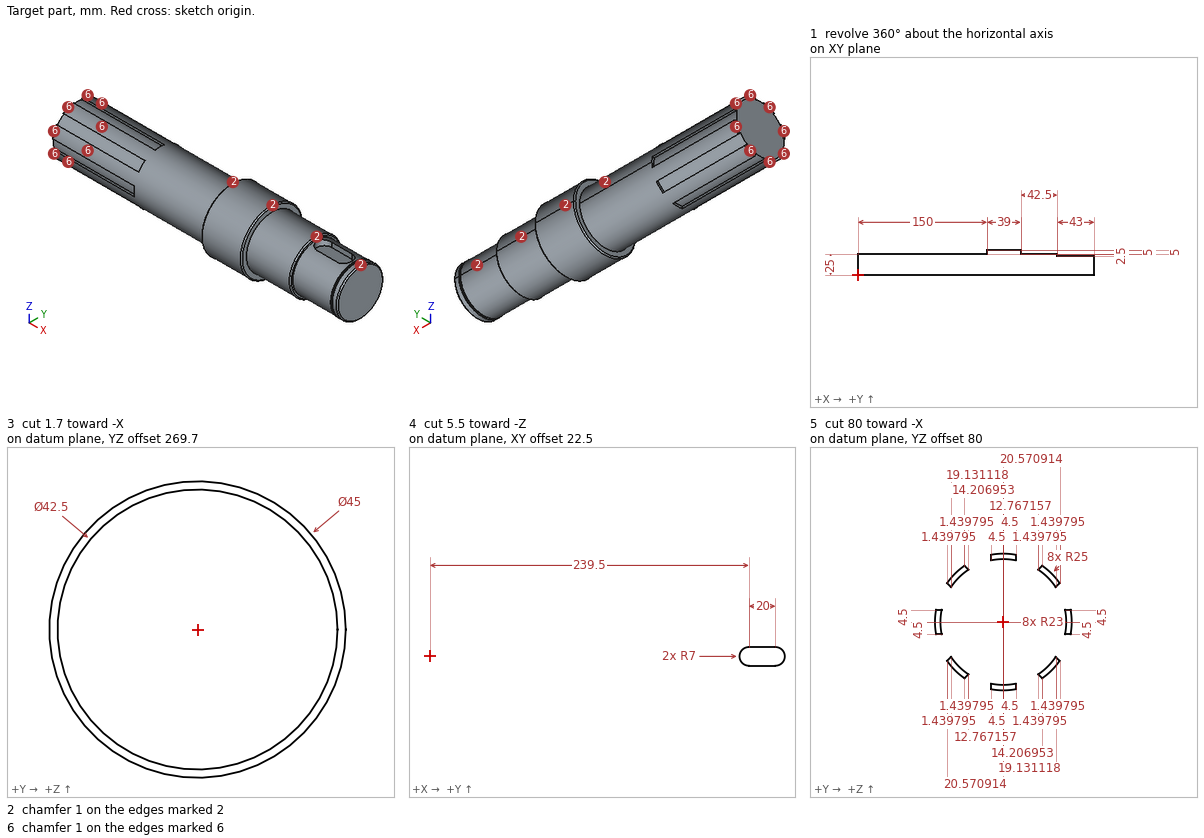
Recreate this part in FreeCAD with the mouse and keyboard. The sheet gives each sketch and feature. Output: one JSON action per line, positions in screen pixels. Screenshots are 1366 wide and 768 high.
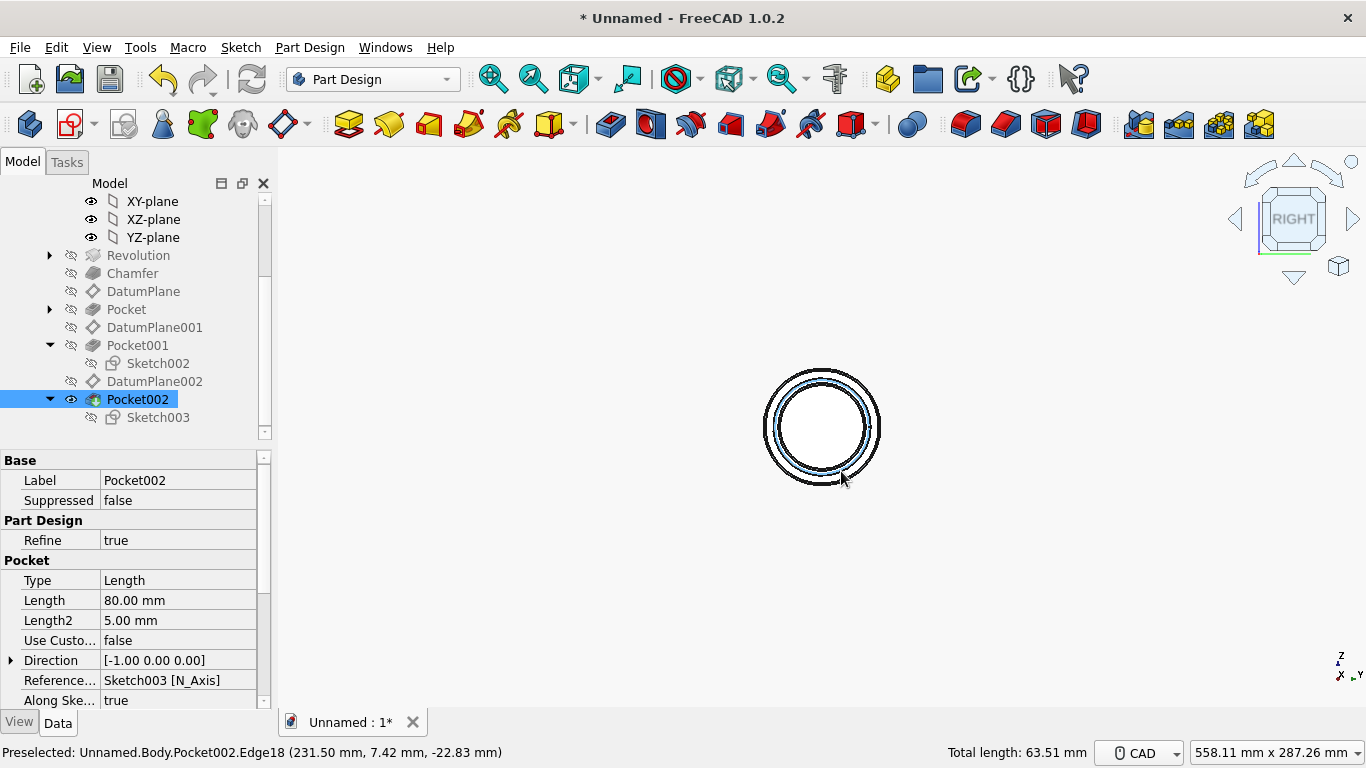
{"action": "key", "text": "5"}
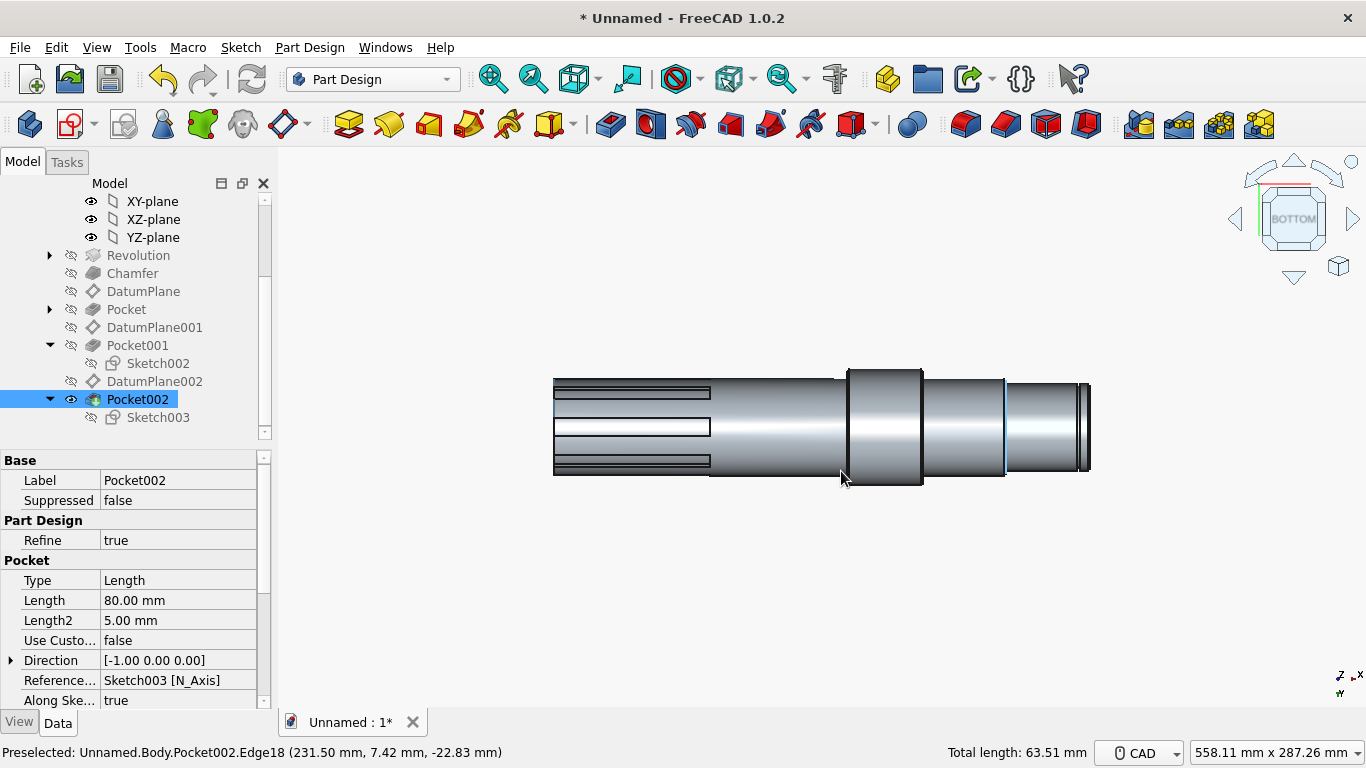
{"action": "left_click", "coordinate": [554, 445], "text": "ctrl"}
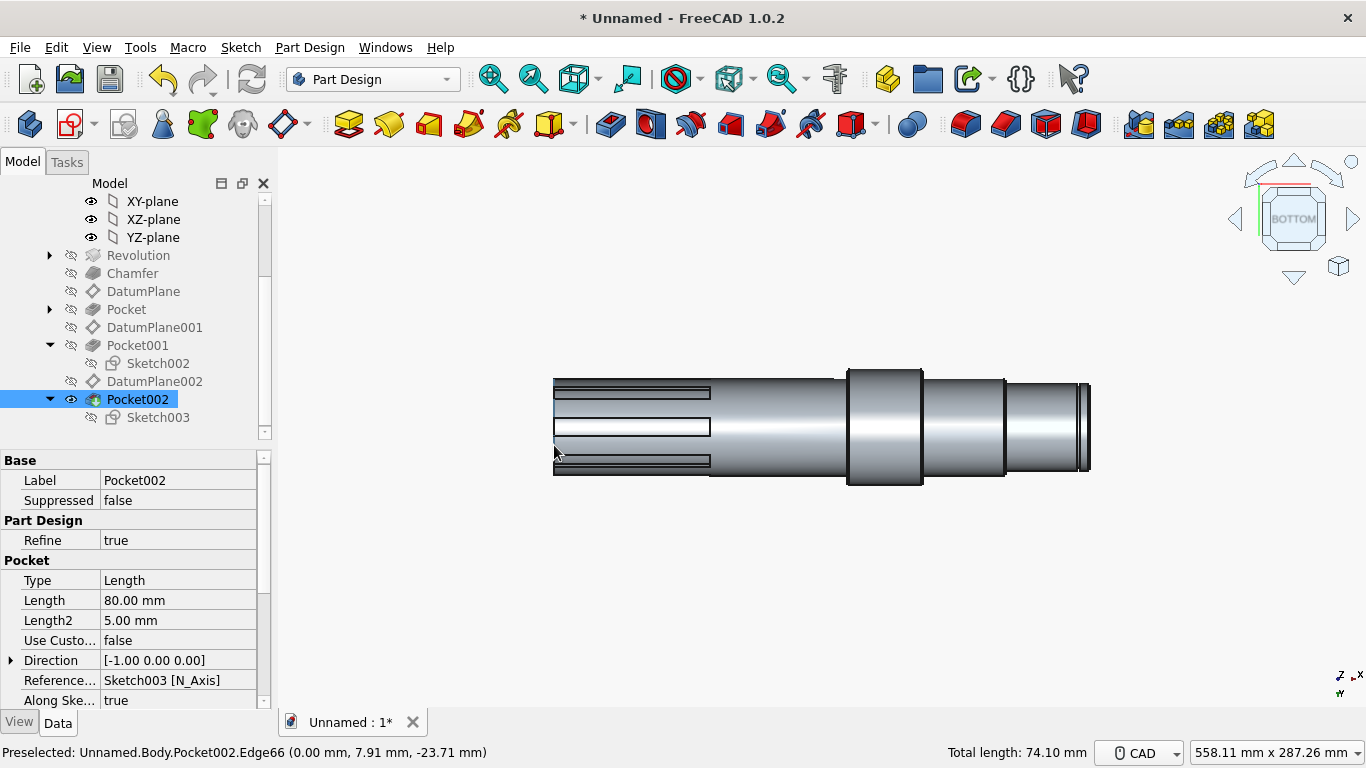
{"action": "left_click", "coordinate": [554, 473], "text": "ctrl"}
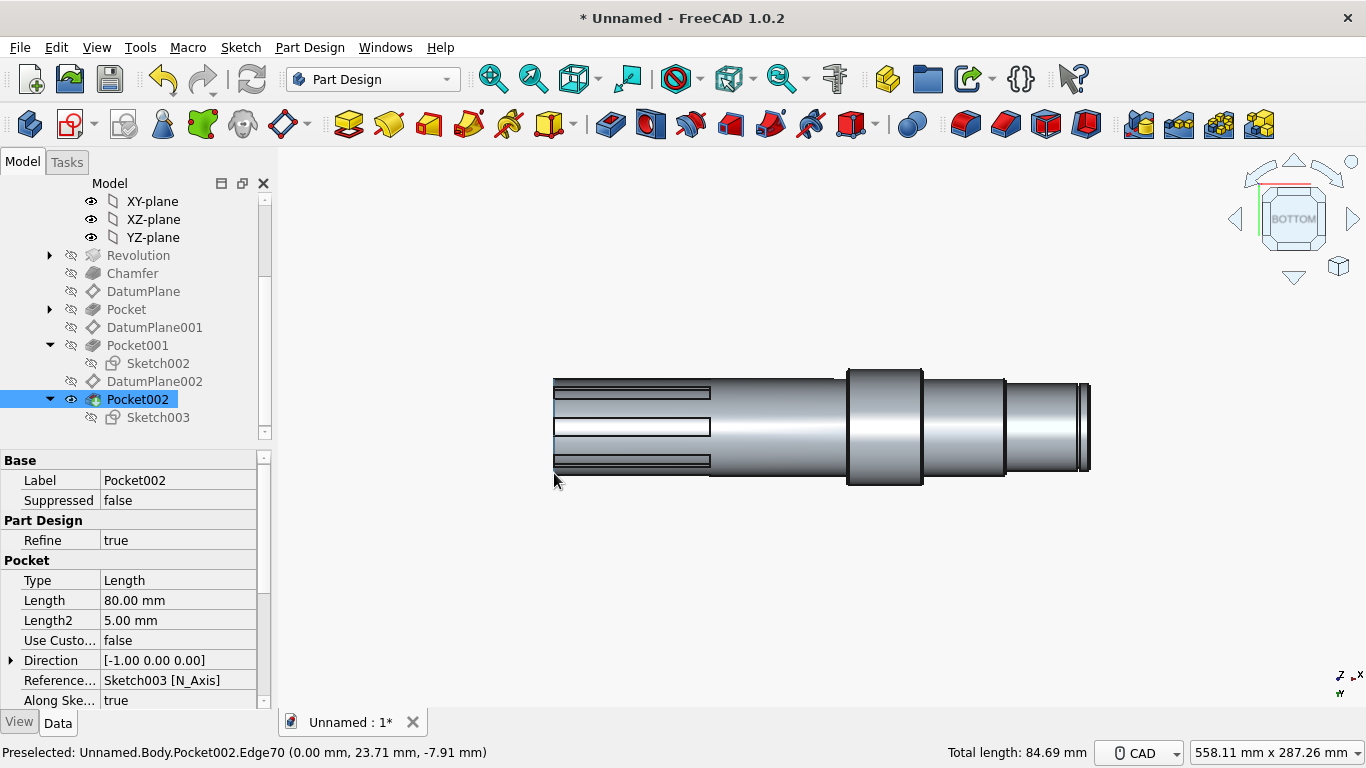
{"action": "left_click", "coordinate": [1006, 124]}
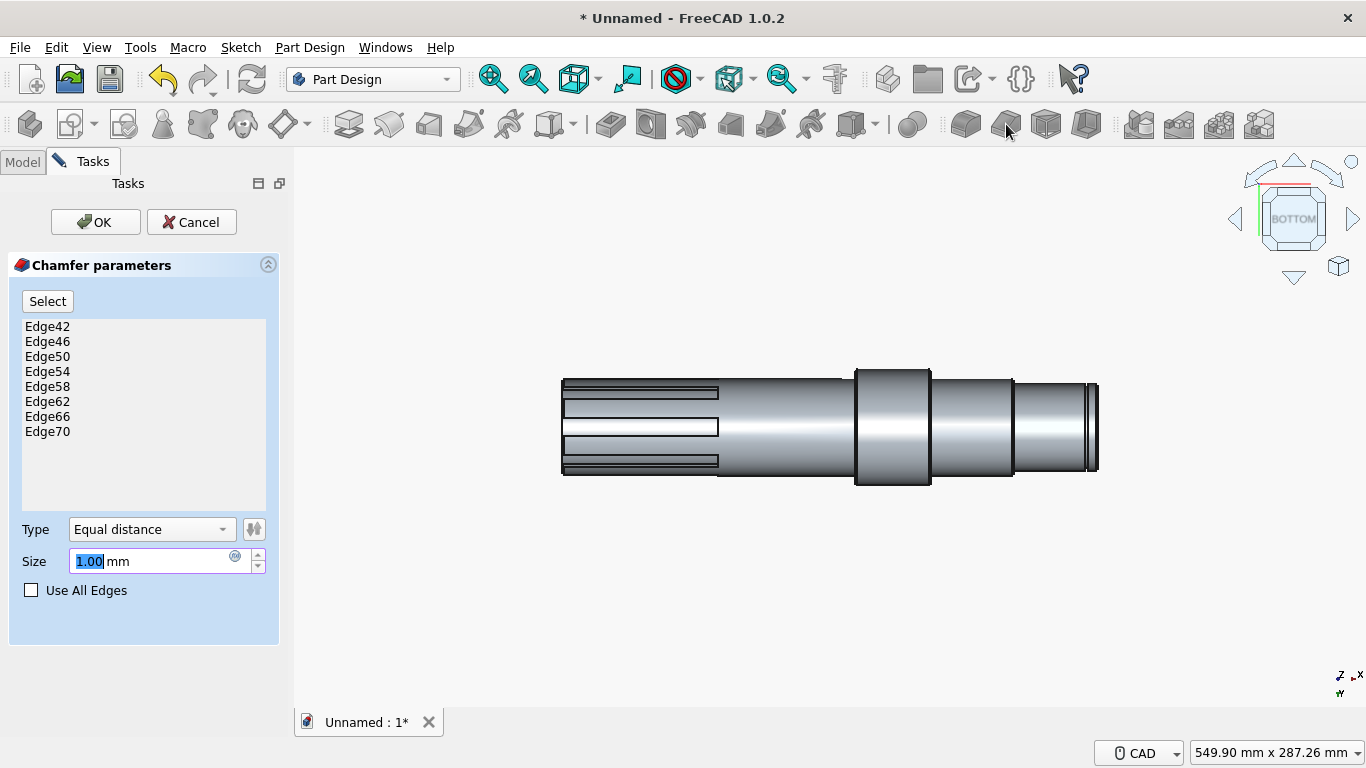
{"action": "type", "text": "1"}
{"action": "key", "text": "Tab"}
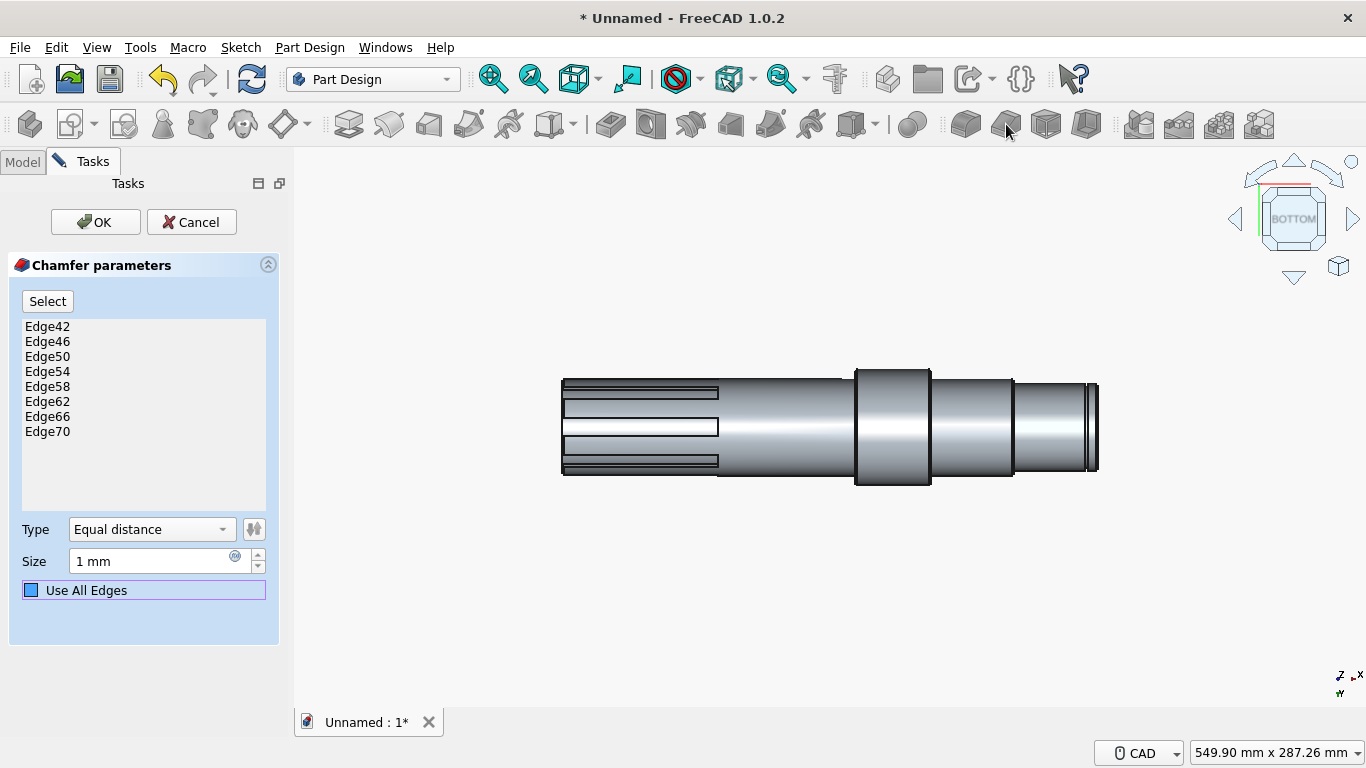
{"action": "left_click", "coordinate": [96, 222]}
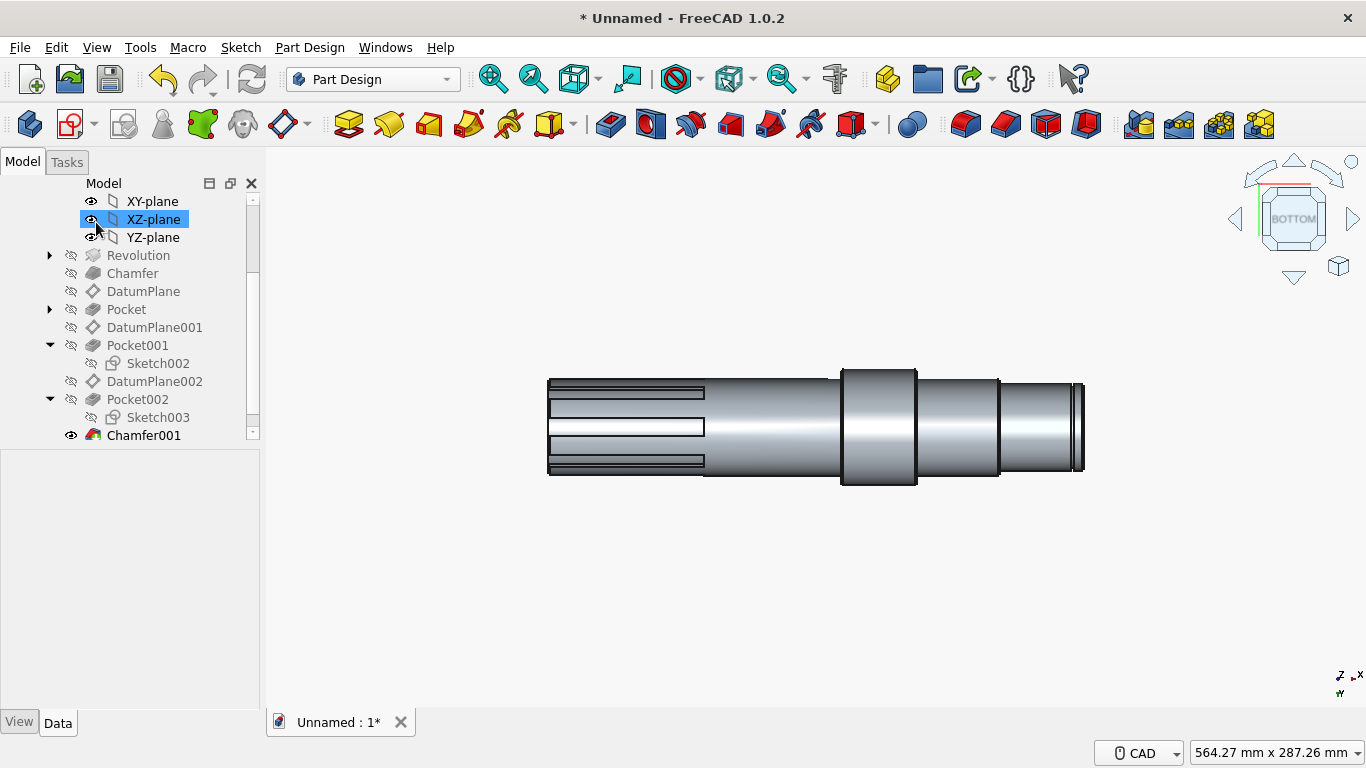
{"action": "key", "text": "0"}